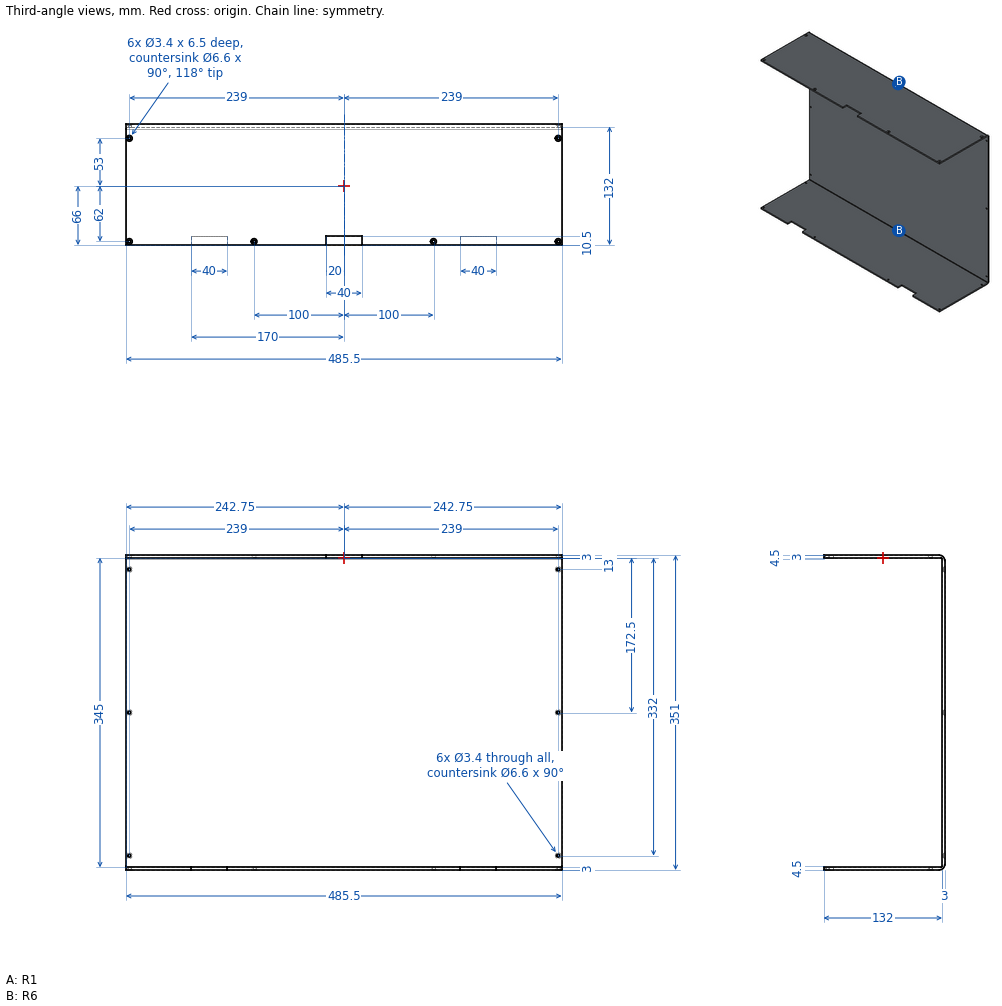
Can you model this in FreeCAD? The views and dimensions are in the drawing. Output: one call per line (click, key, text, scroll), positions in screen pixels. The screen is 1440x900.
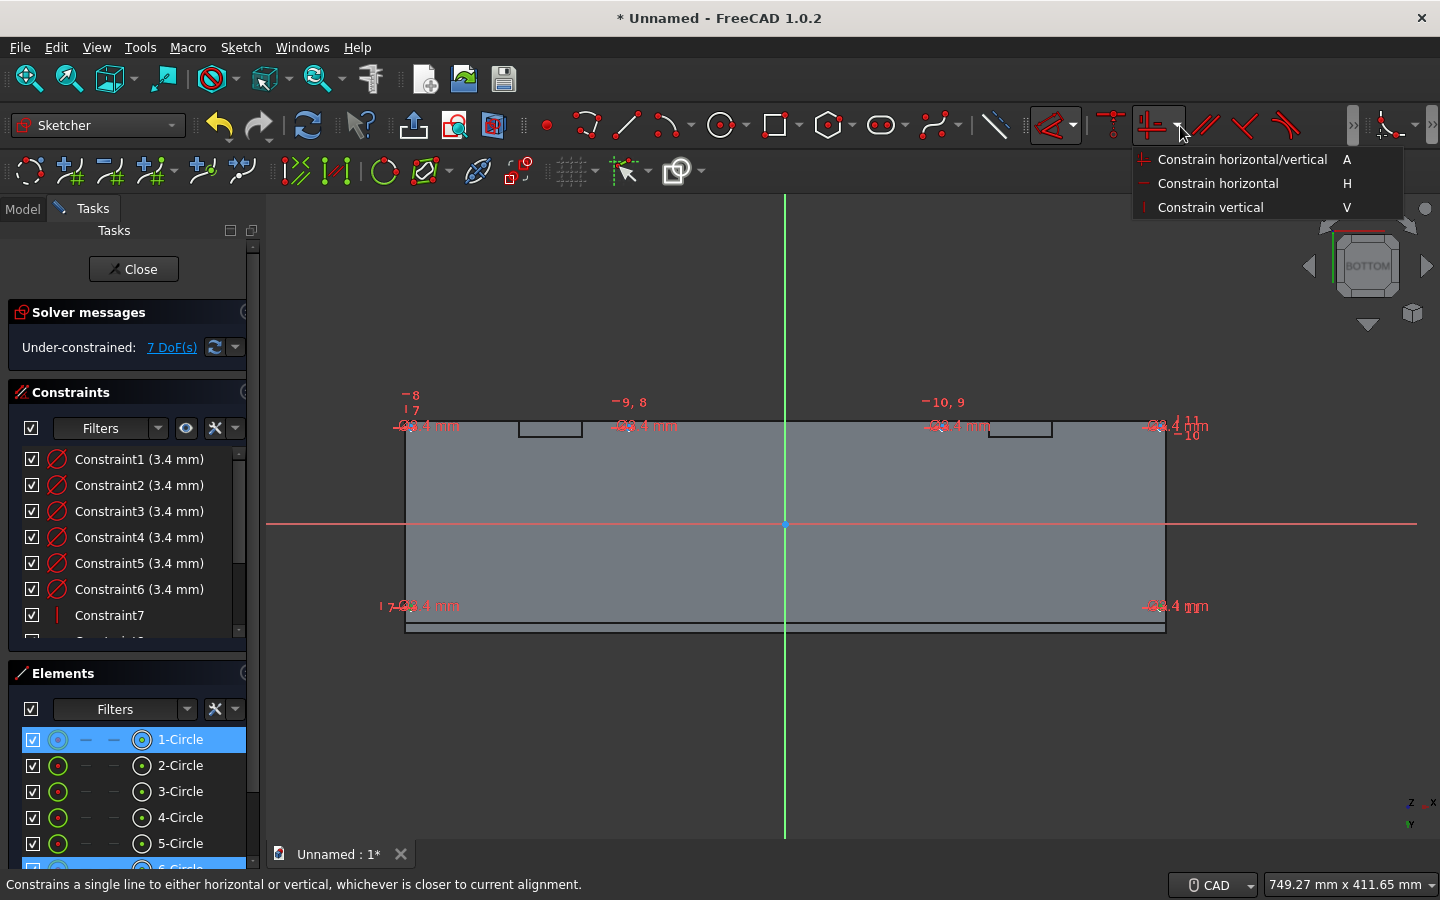
click(1268, 183)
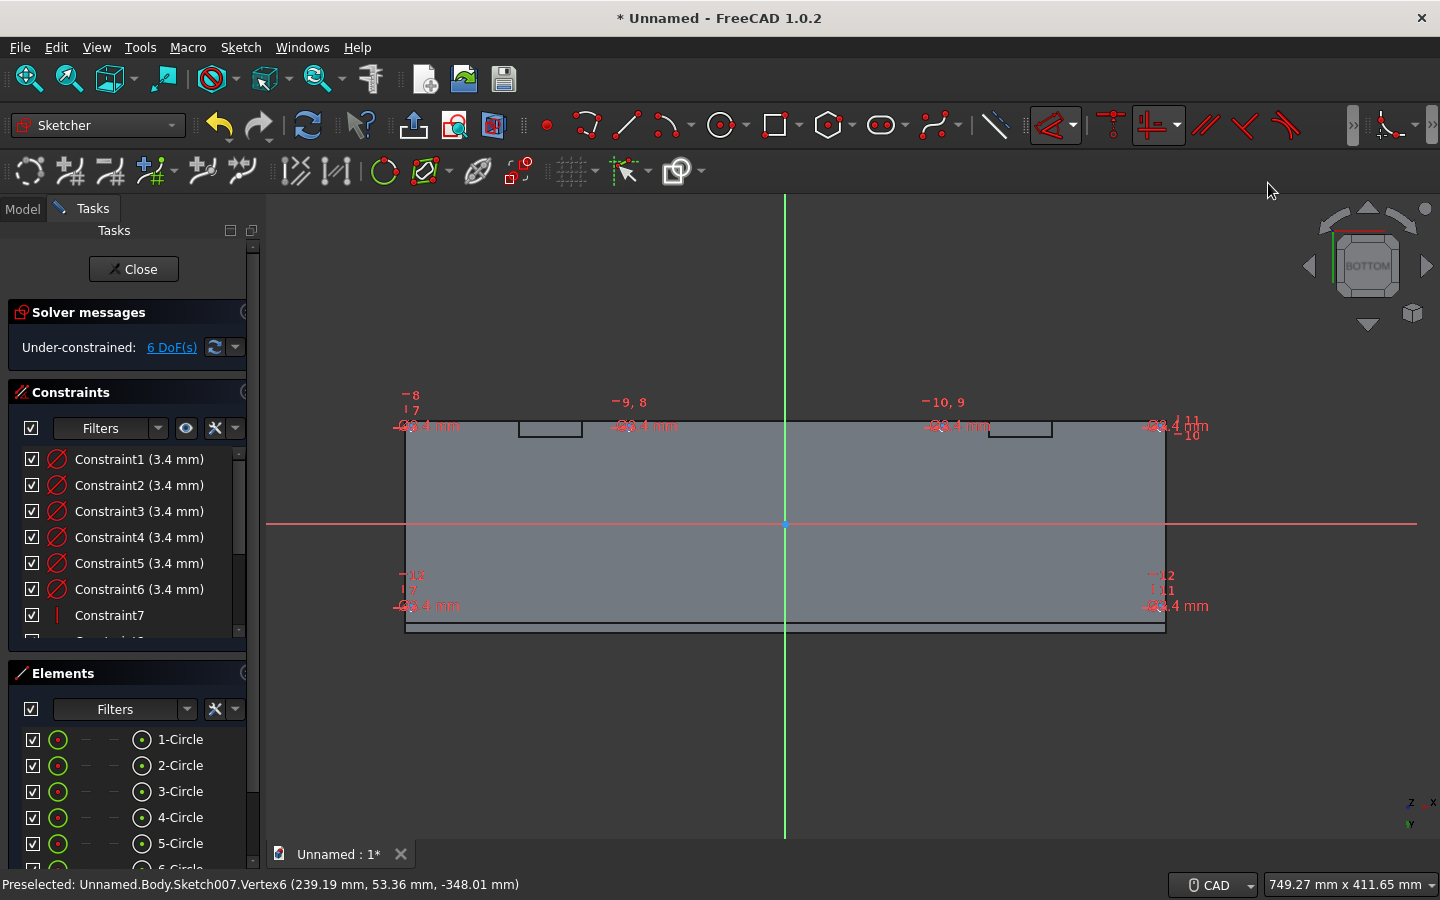
click(411, 608)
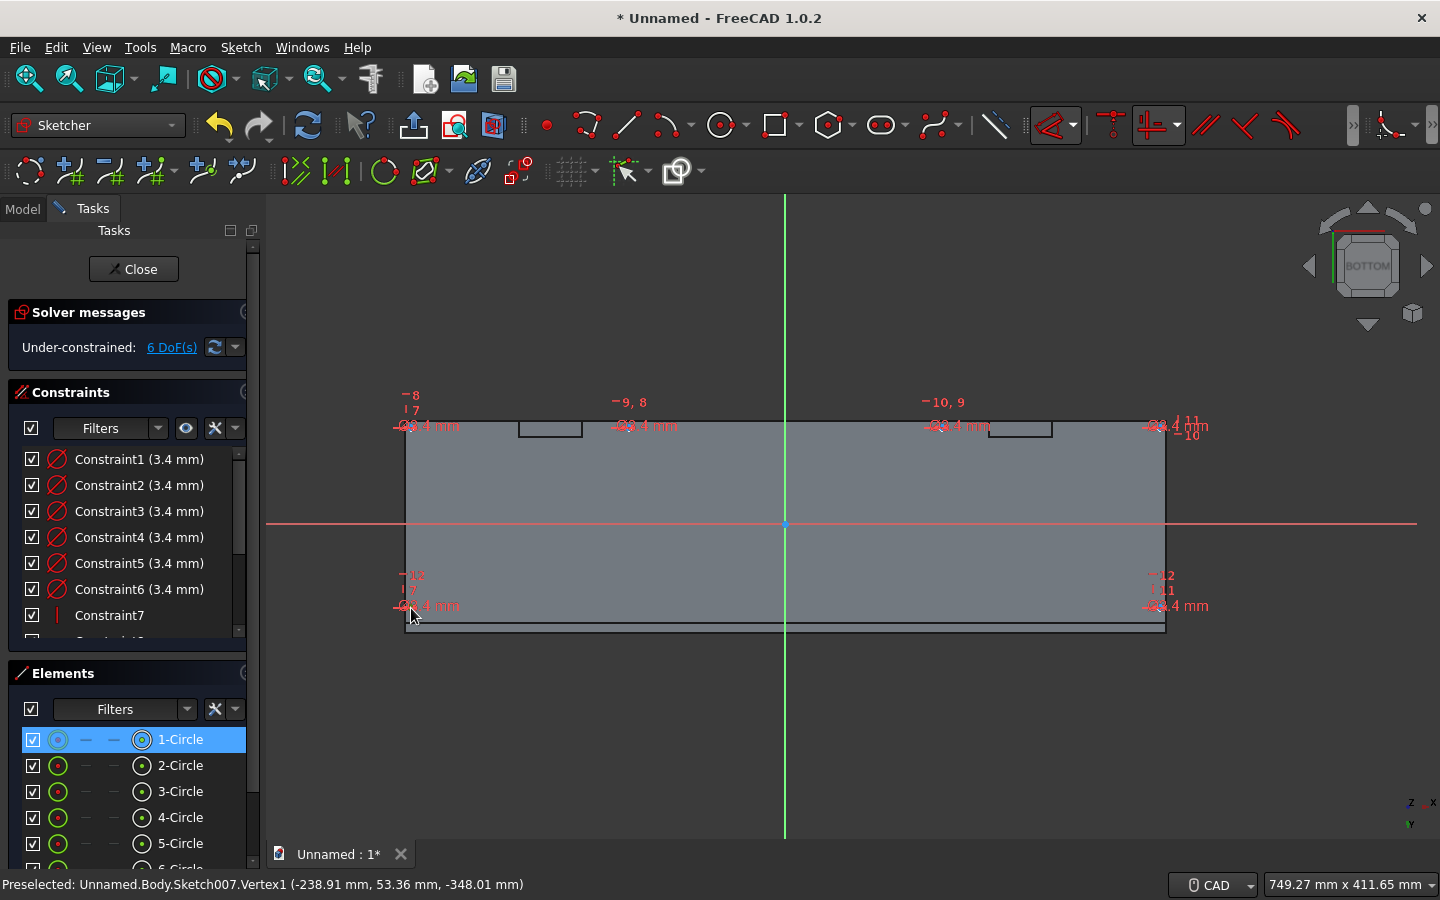
click(1076, 126)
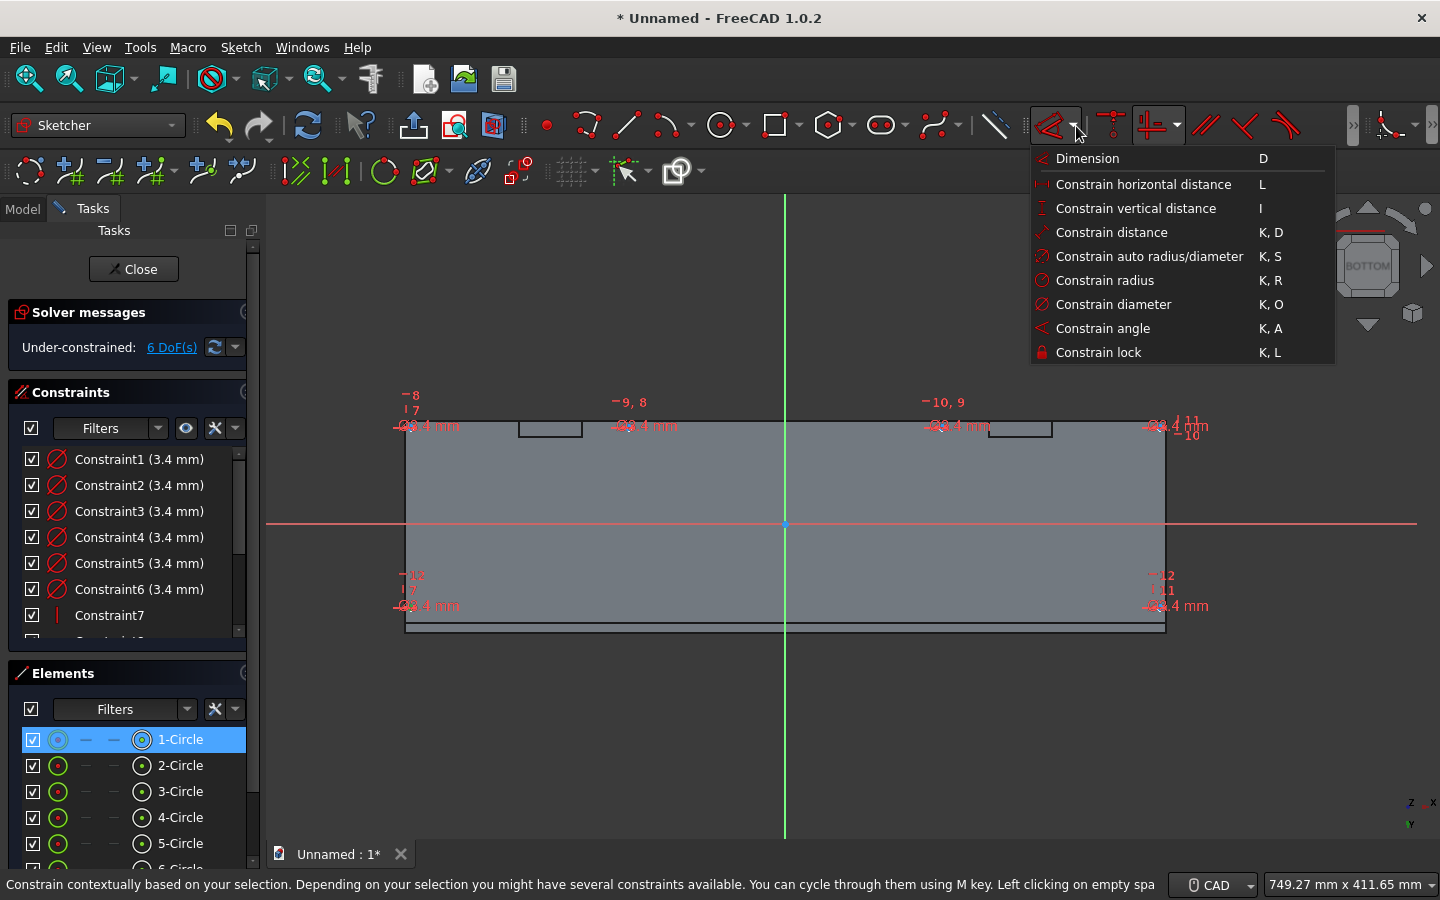
click(1183, 208)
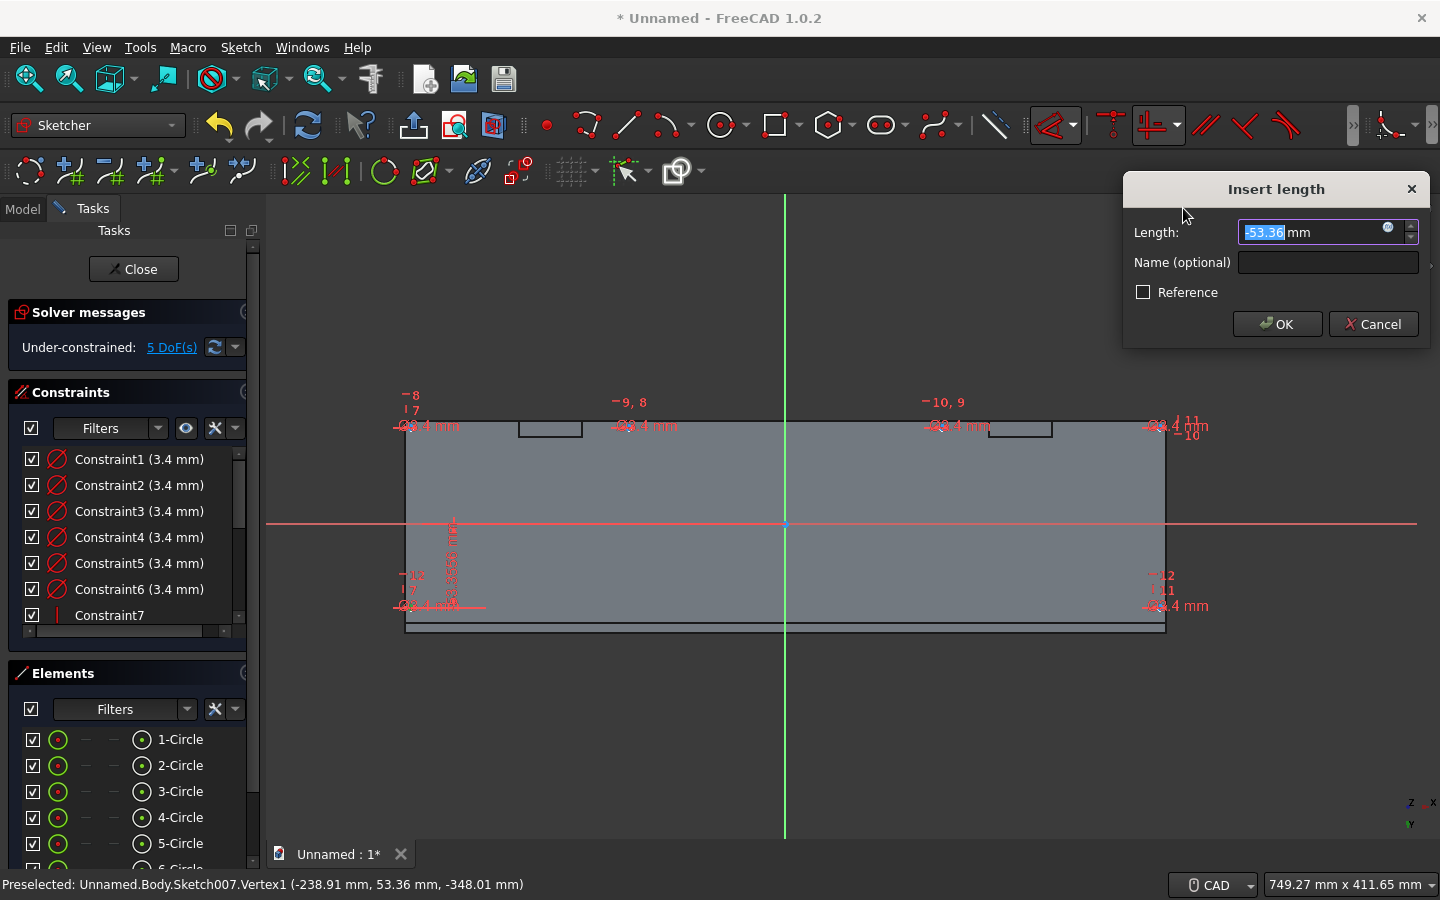
text(-53)
key(Return)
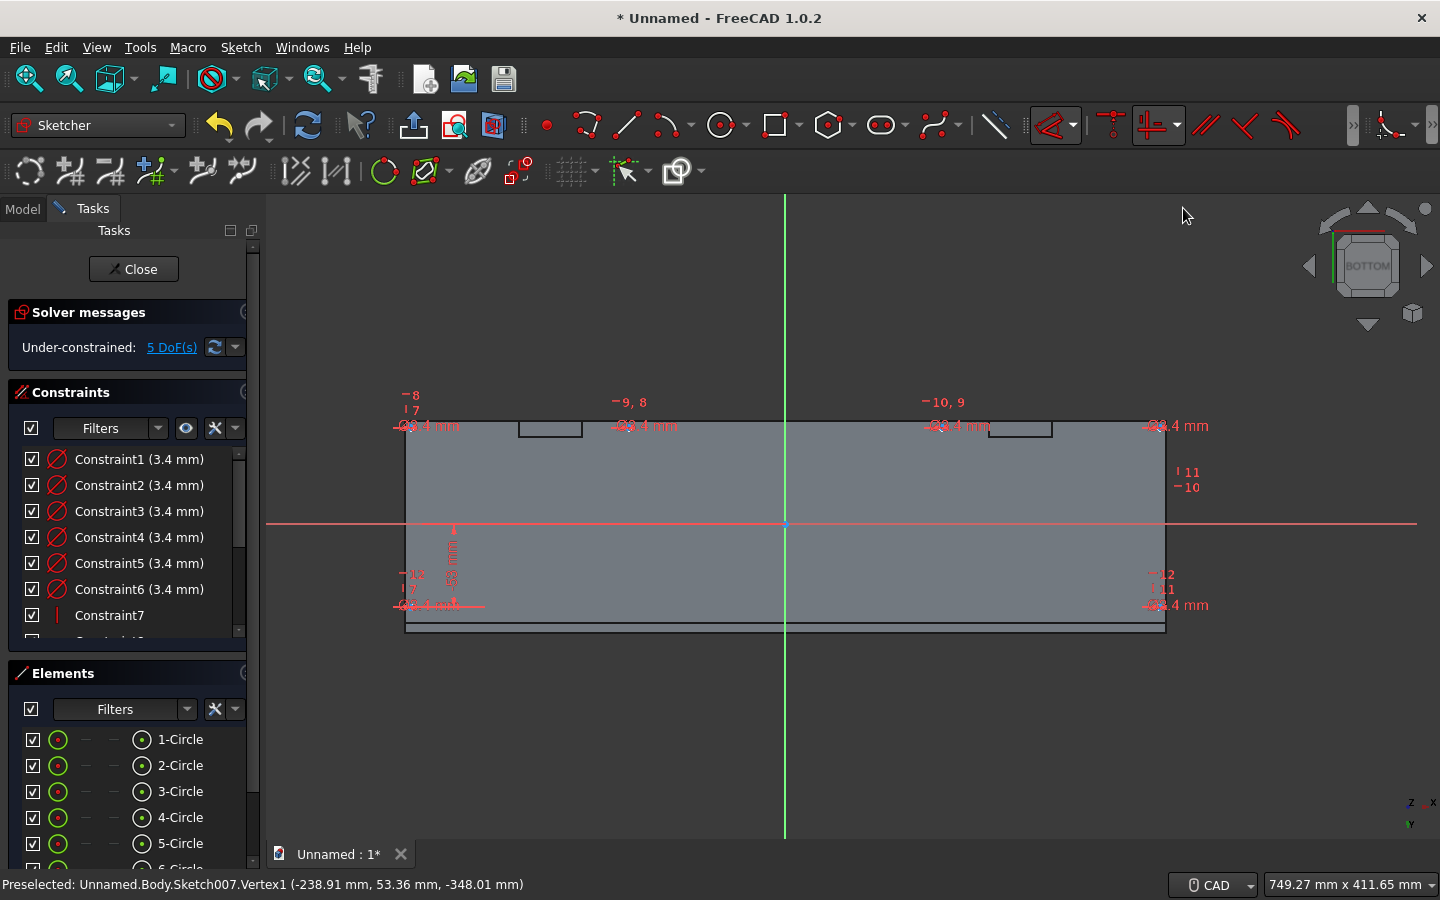
click(411, 428)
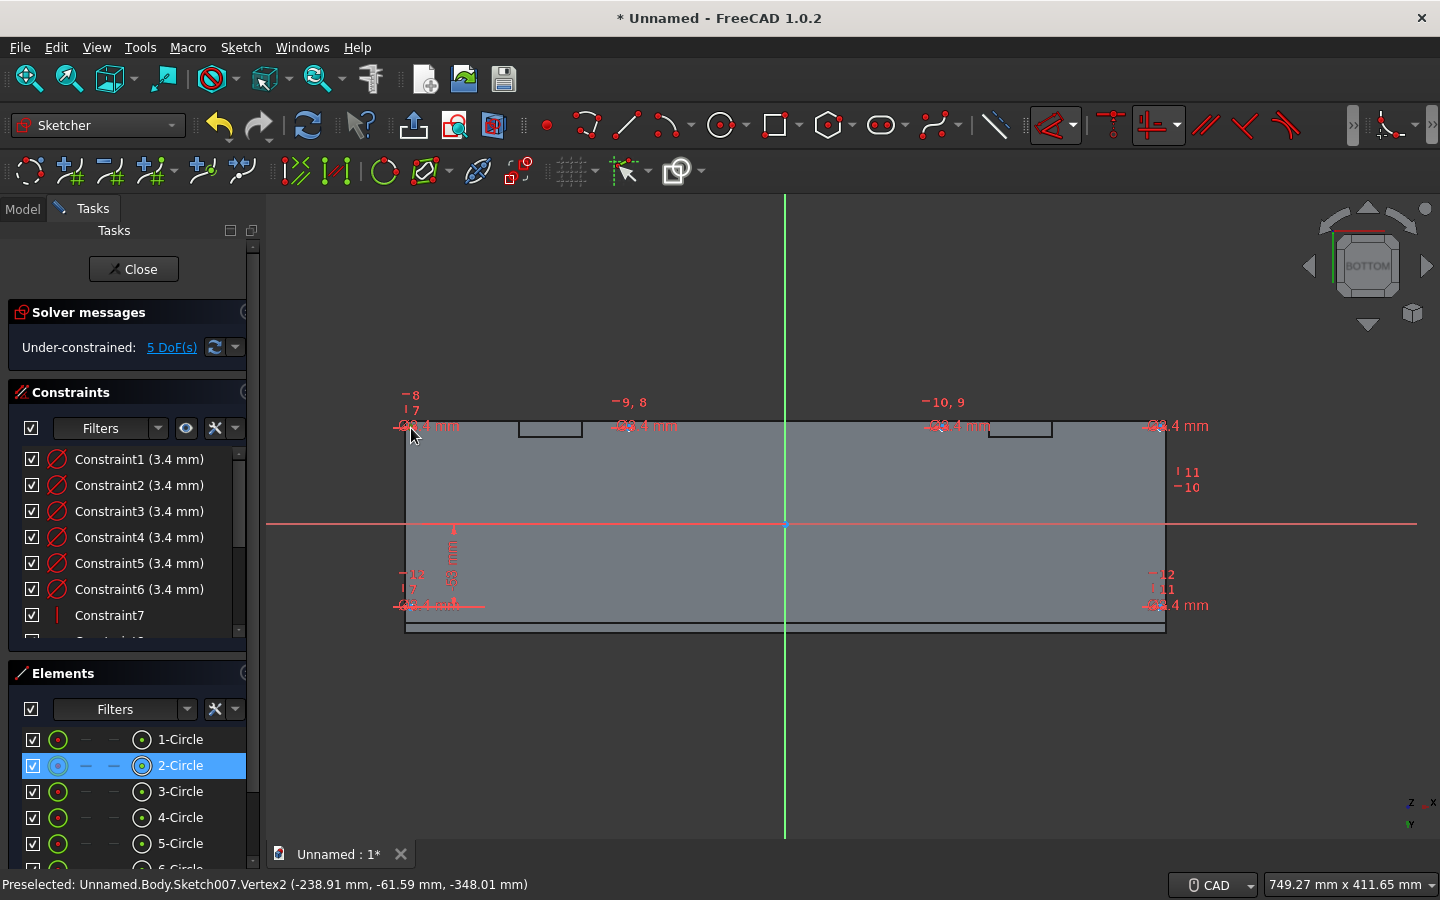
click(1076, 126)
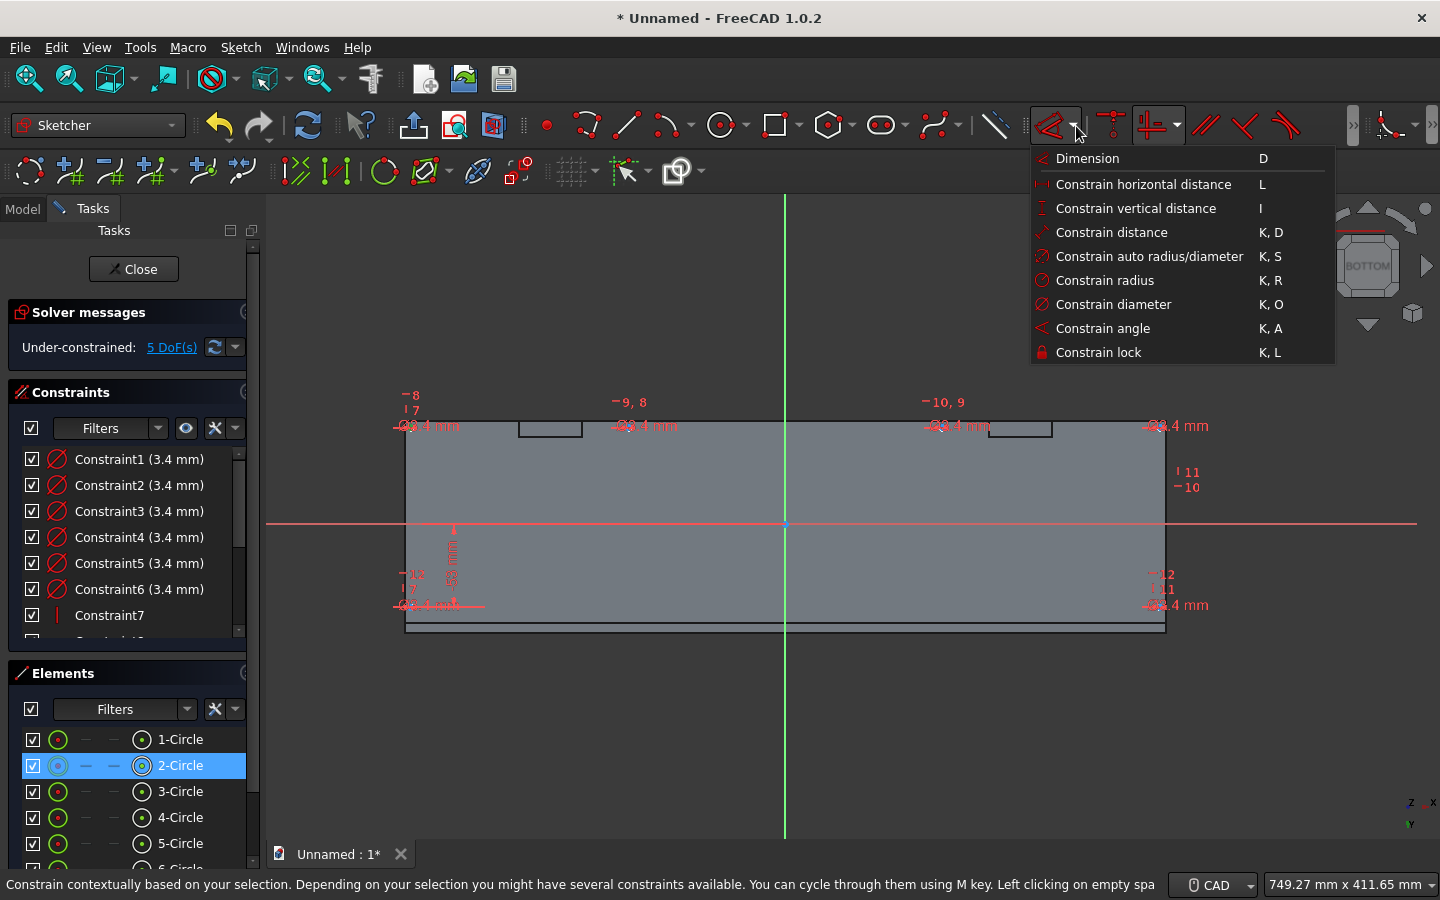
click(1183, 208)